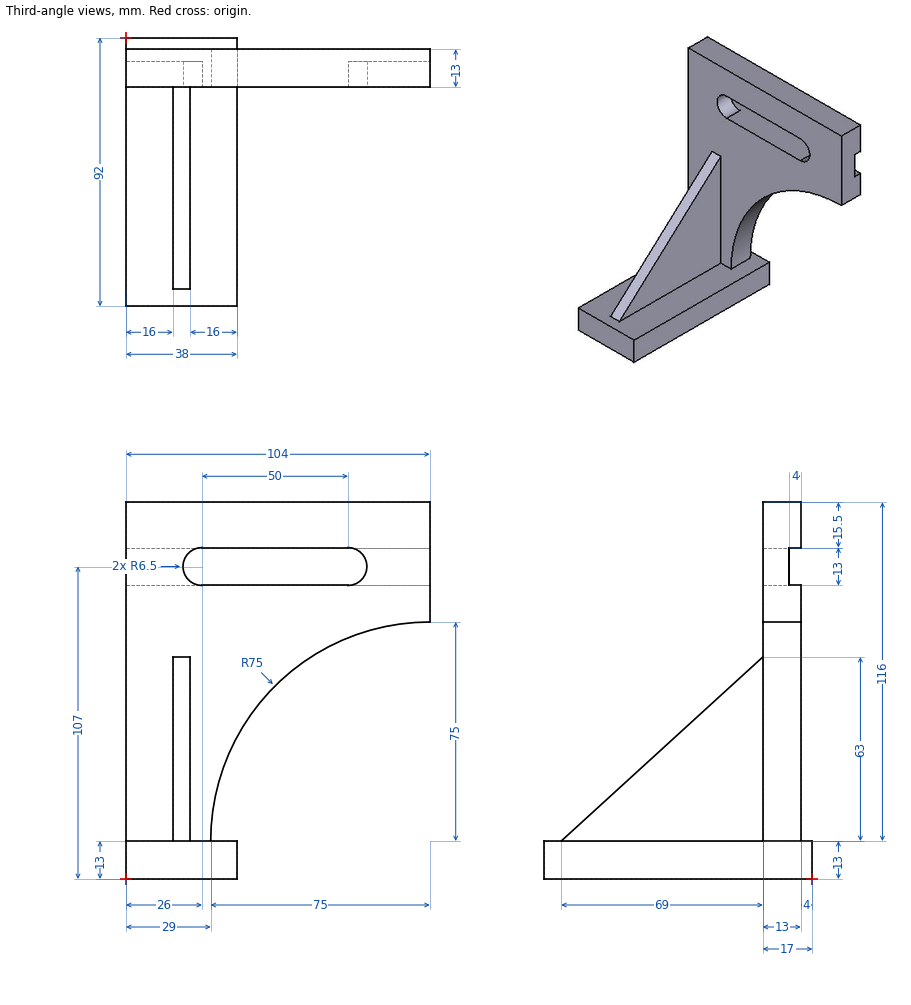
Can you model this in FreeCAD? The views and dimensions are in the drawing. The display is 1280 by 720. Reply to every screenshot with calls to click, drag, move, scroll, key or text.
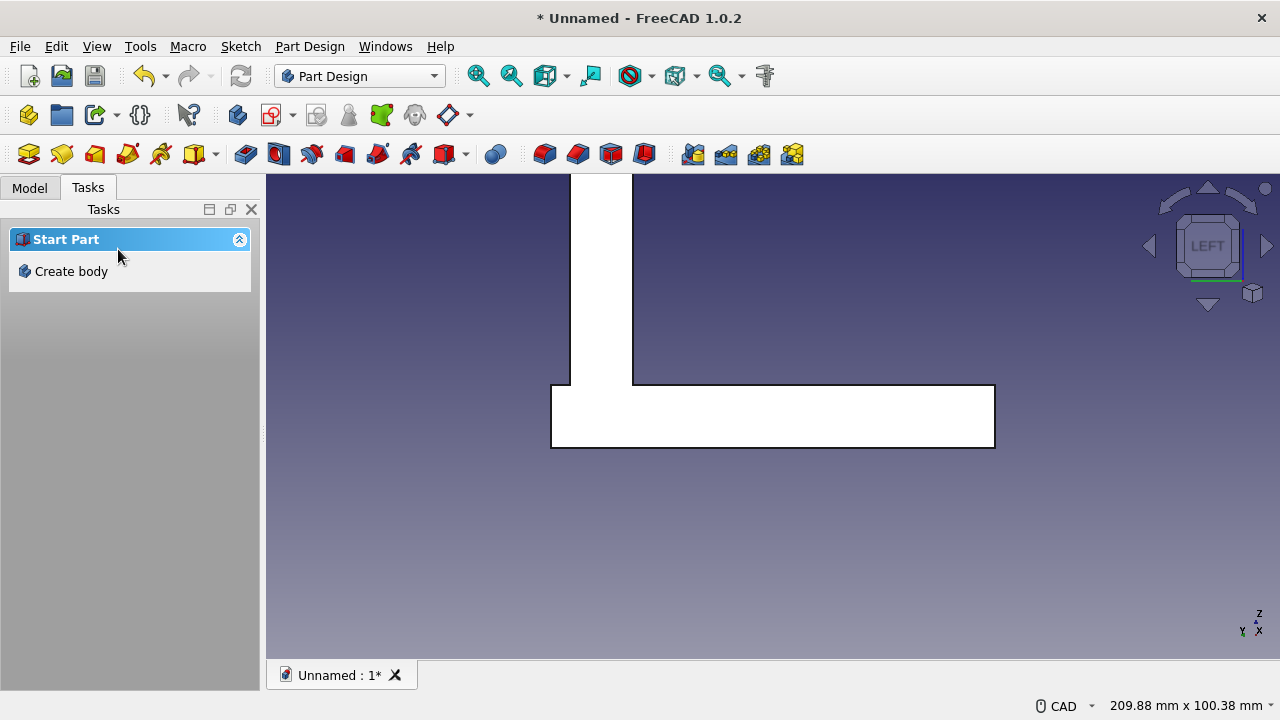
click(479, 76)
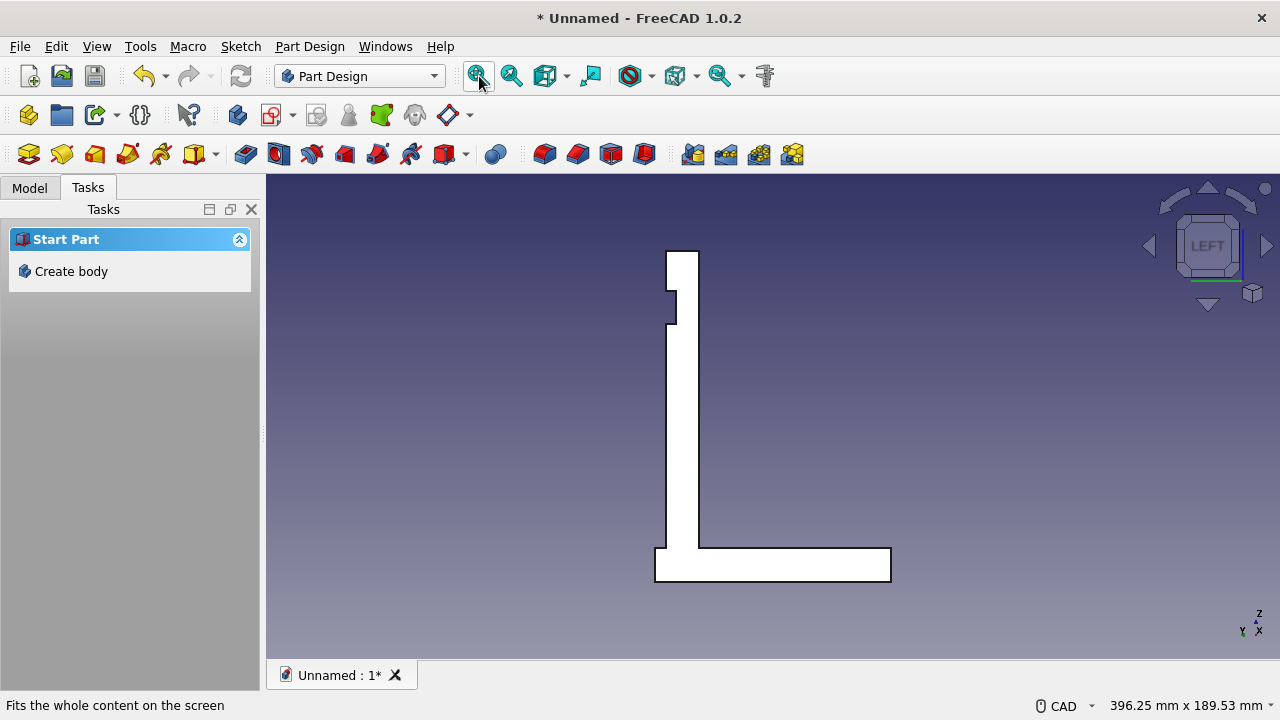
key(0)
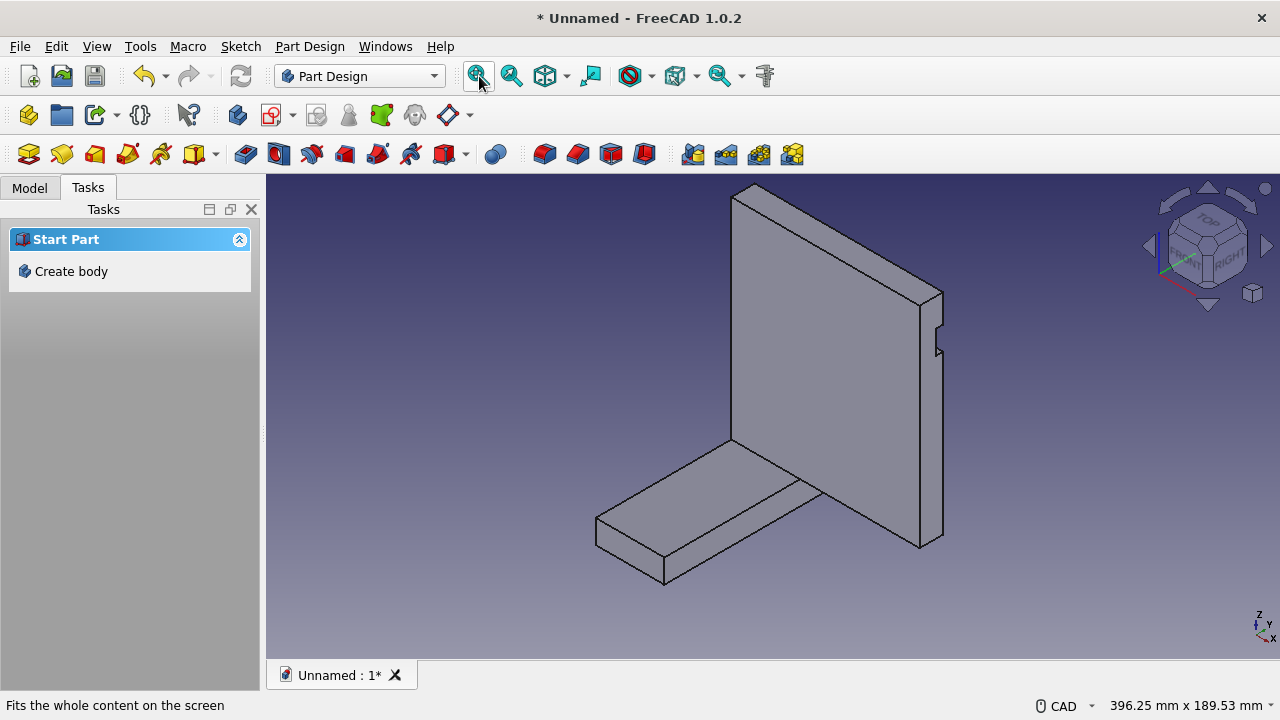
click(825, 372)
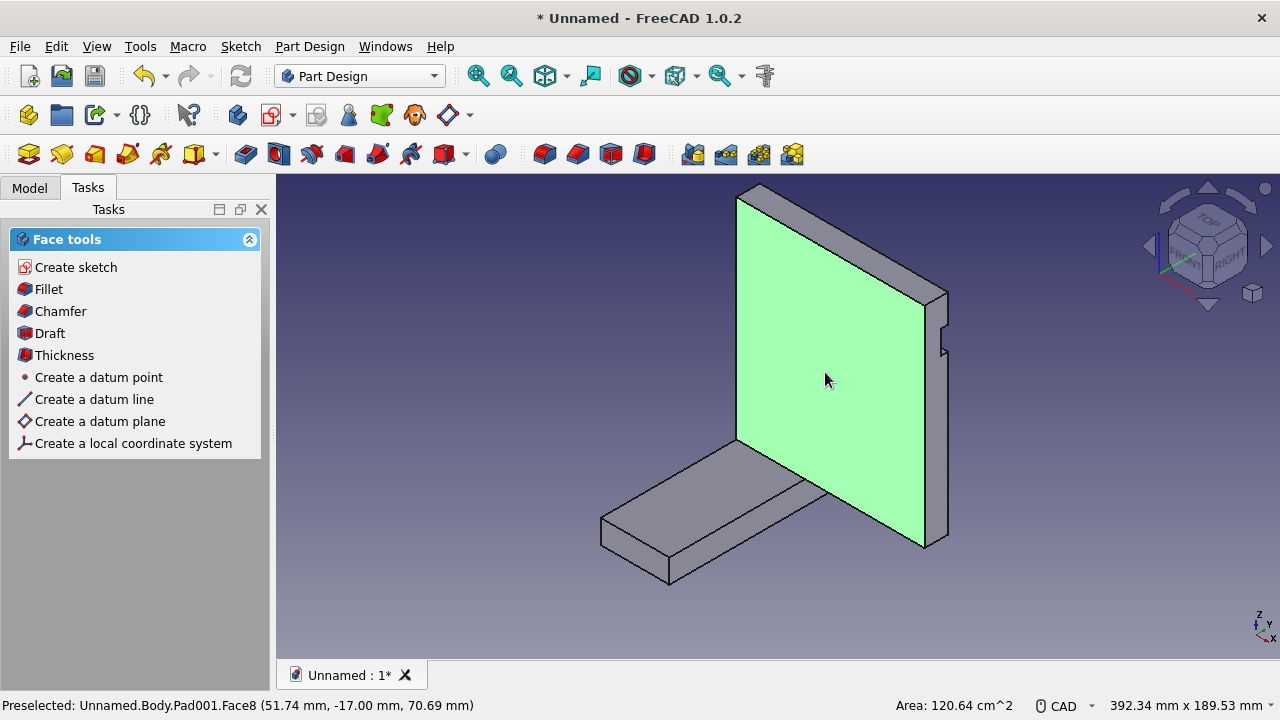
click(270, 116)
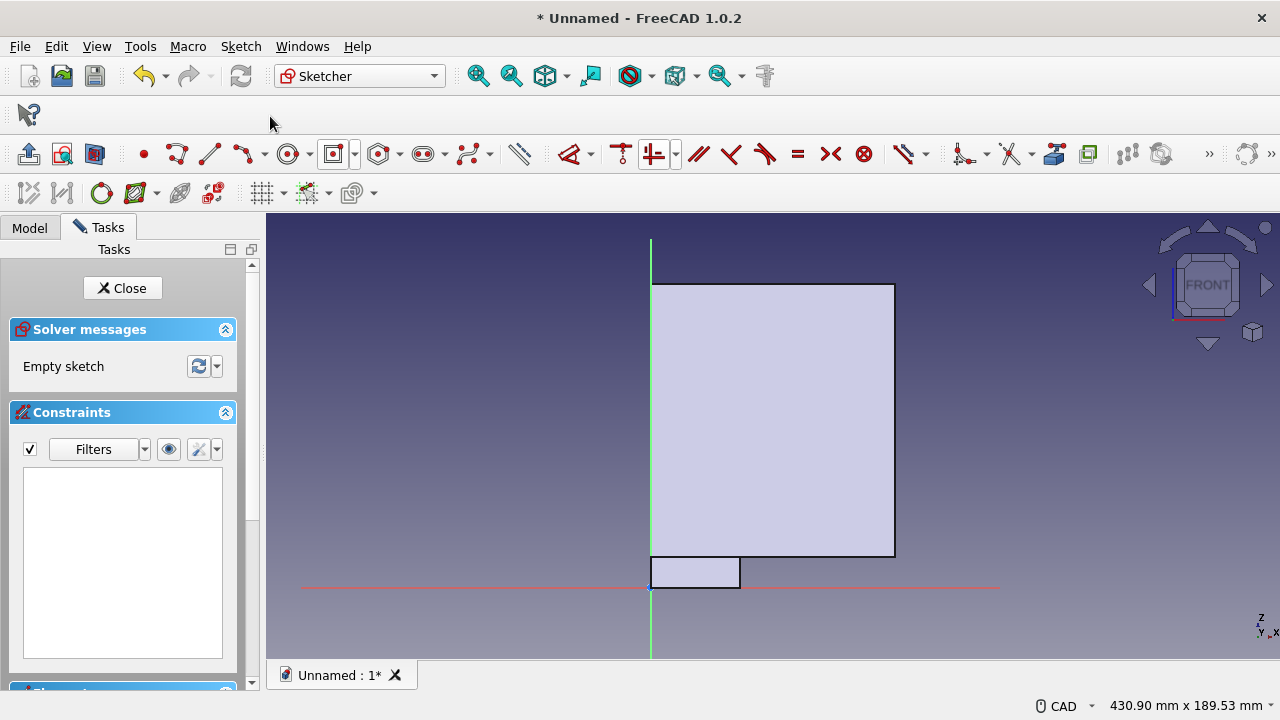
click(177, 154)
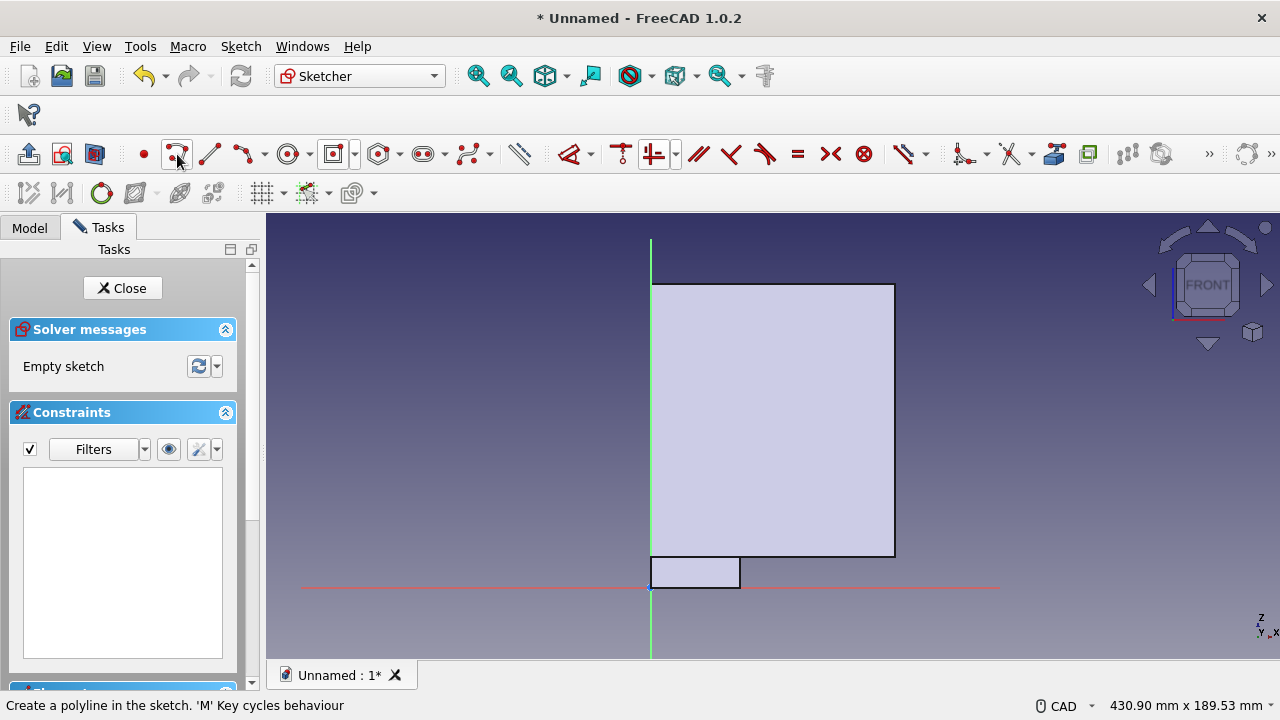
click(719, 557)
click(895, 557)
click(895, 381)
right_click(895, 381)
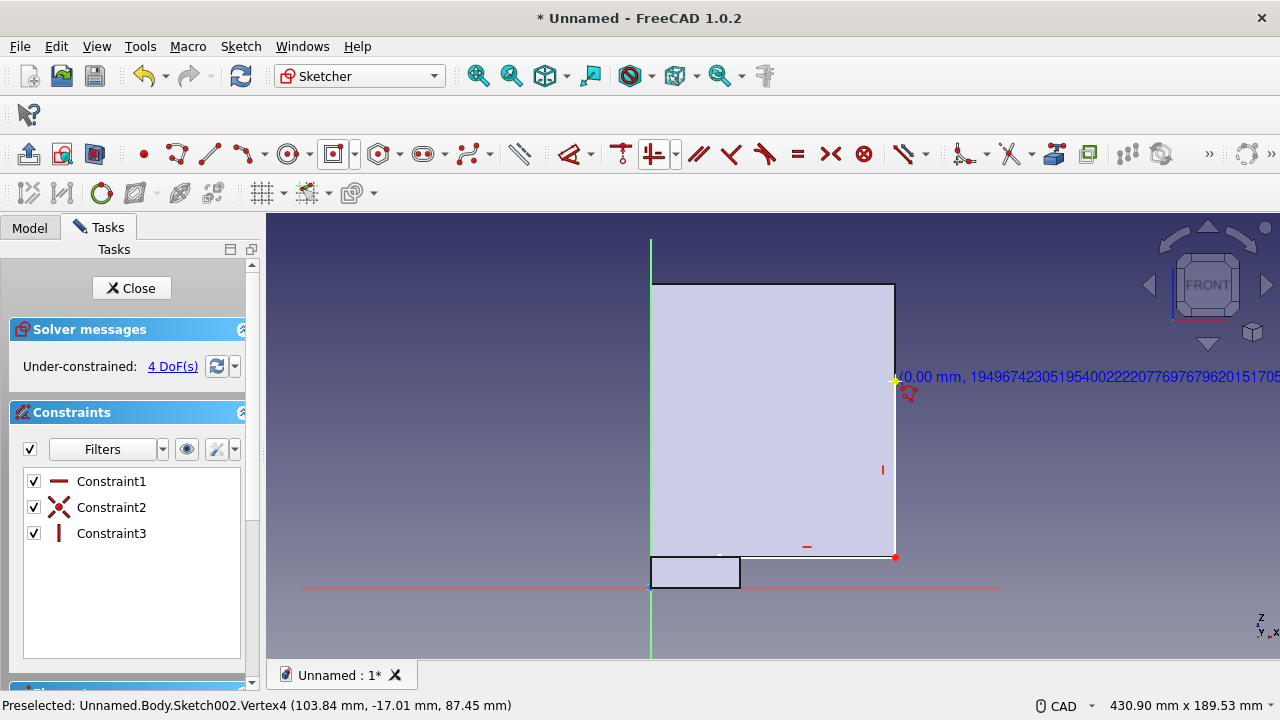
click(242, 154)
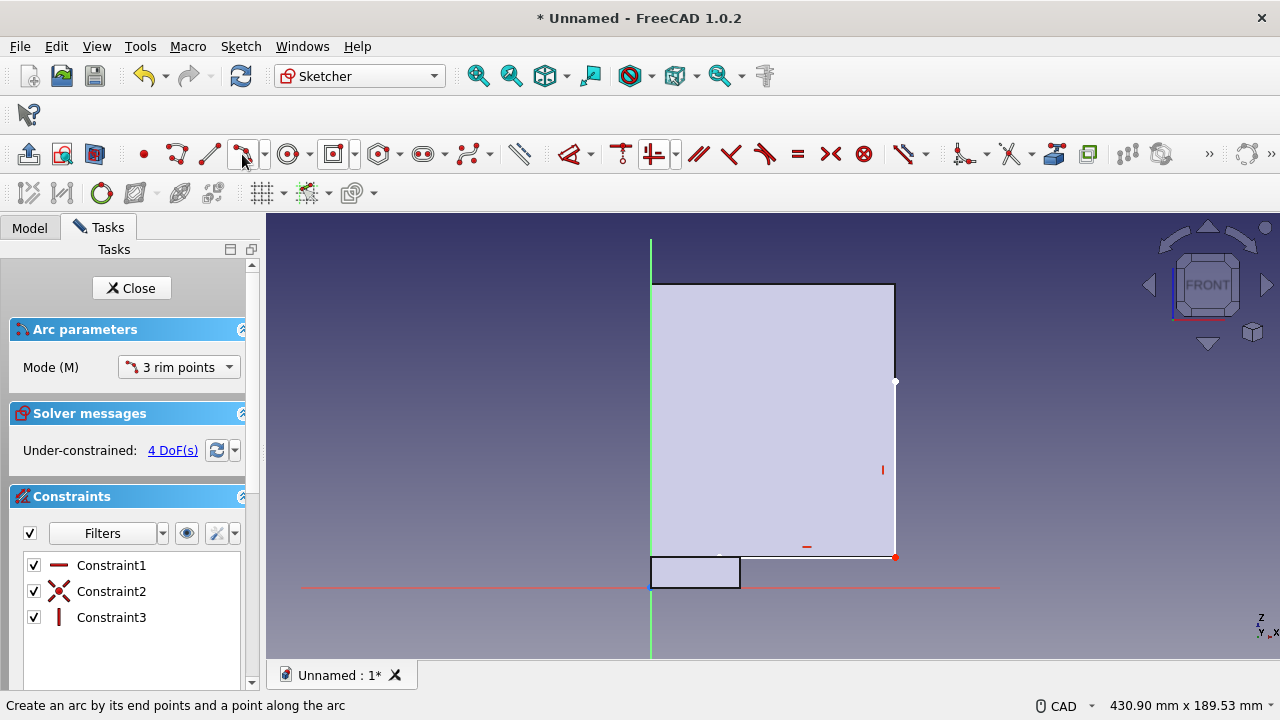
click(895, 382)
click(719, 558)
click(771, 432)
key(Escape)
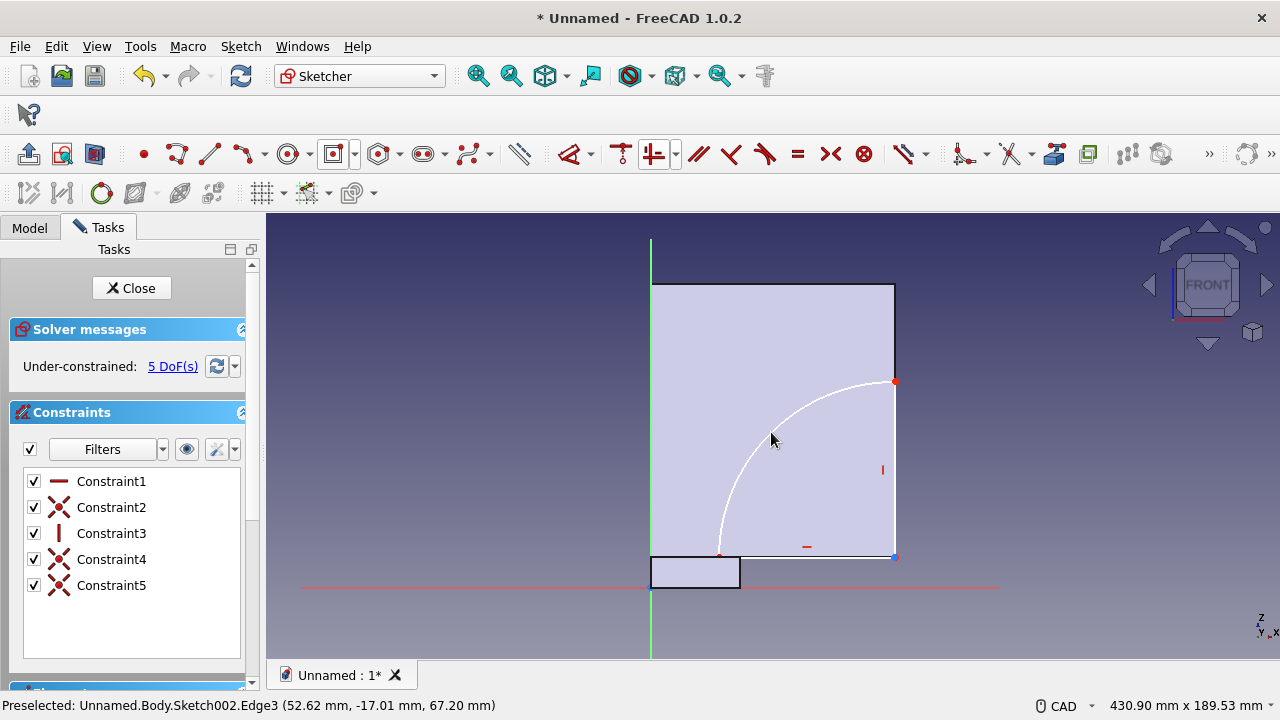
click(568, 154)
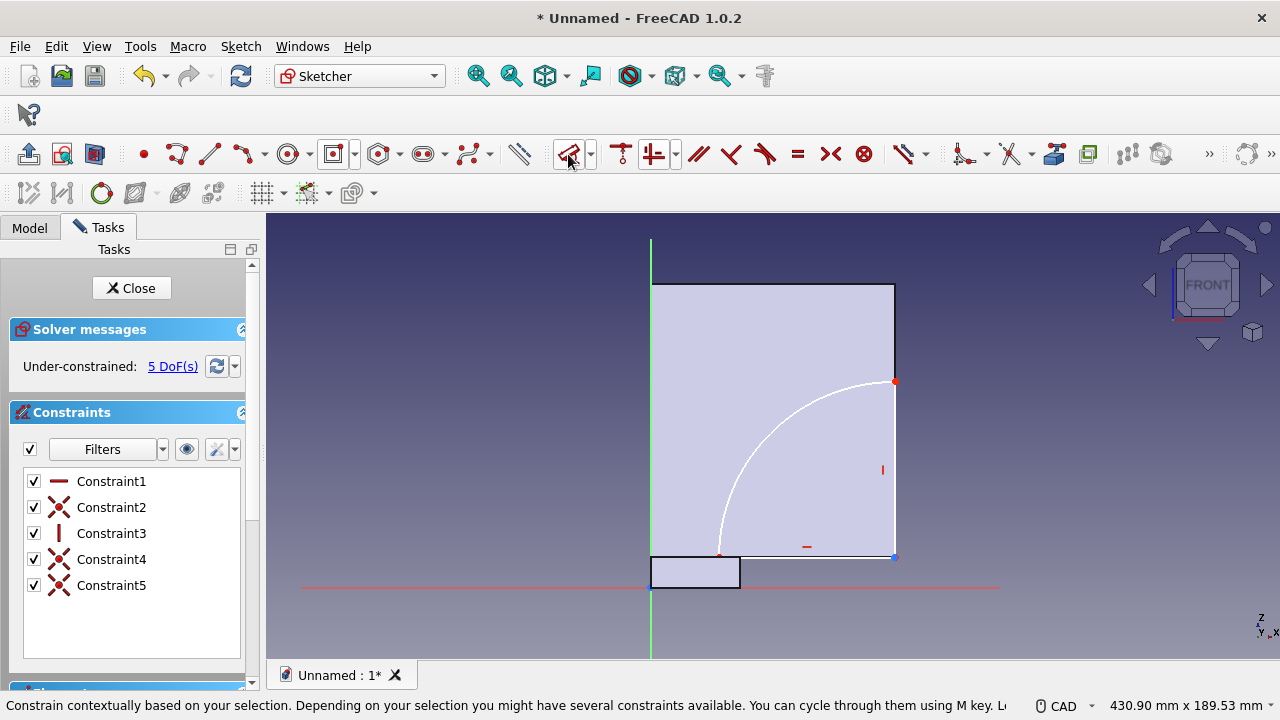
click(815, 401)
click(800, 372)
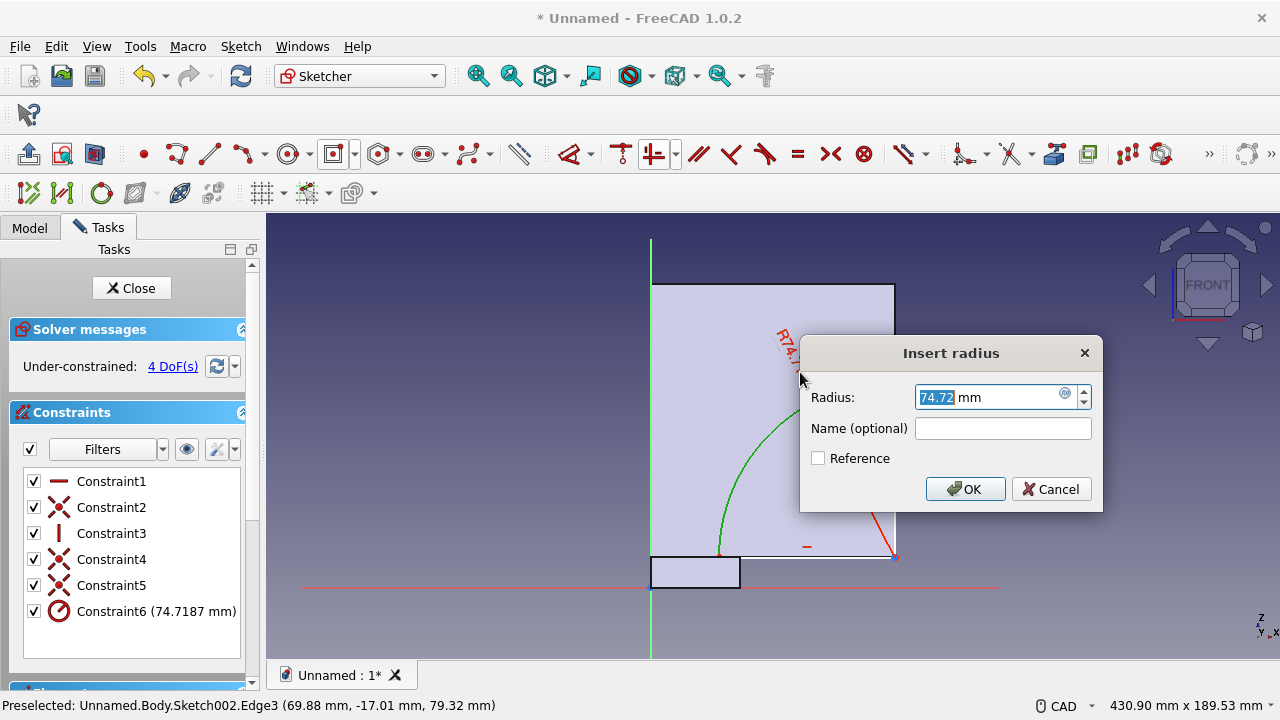
text(75)
key(Return)